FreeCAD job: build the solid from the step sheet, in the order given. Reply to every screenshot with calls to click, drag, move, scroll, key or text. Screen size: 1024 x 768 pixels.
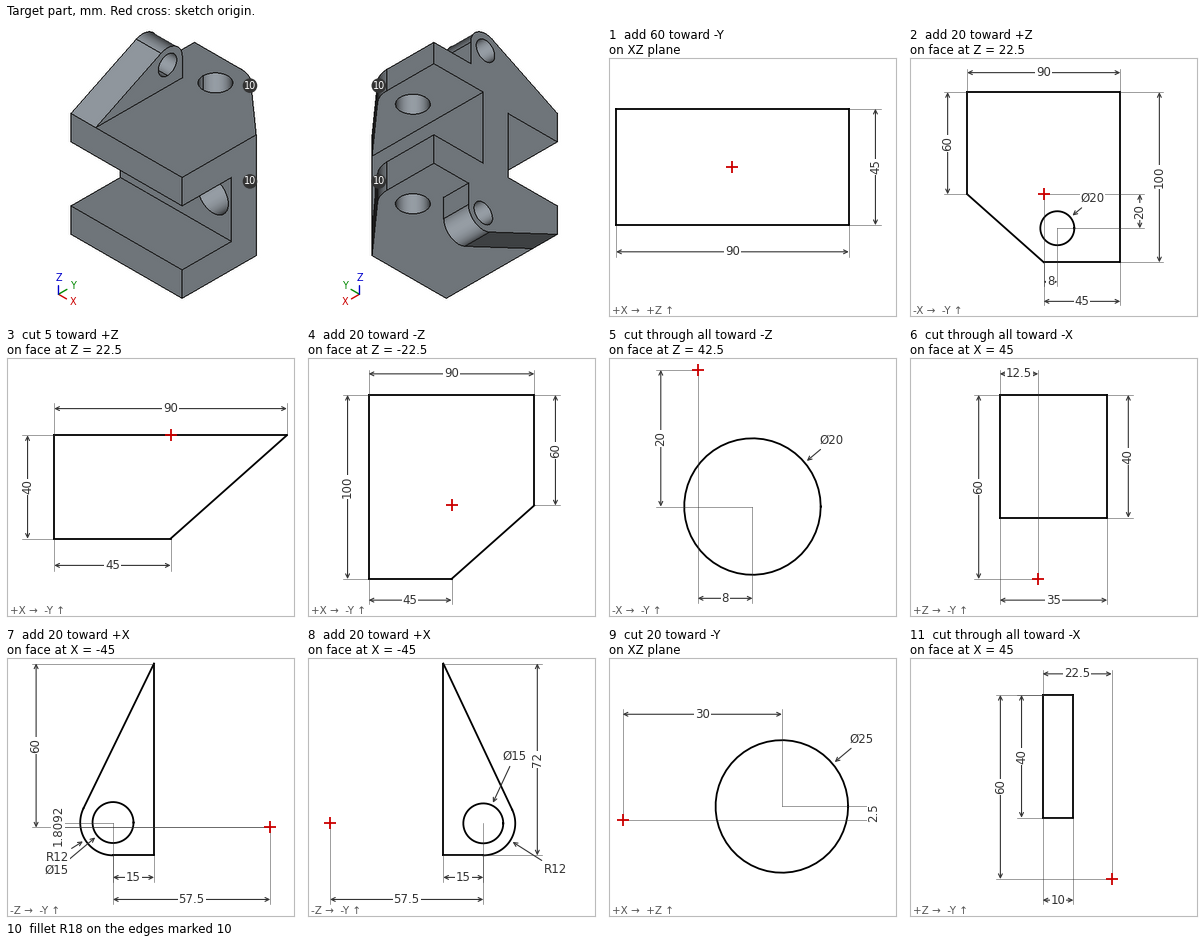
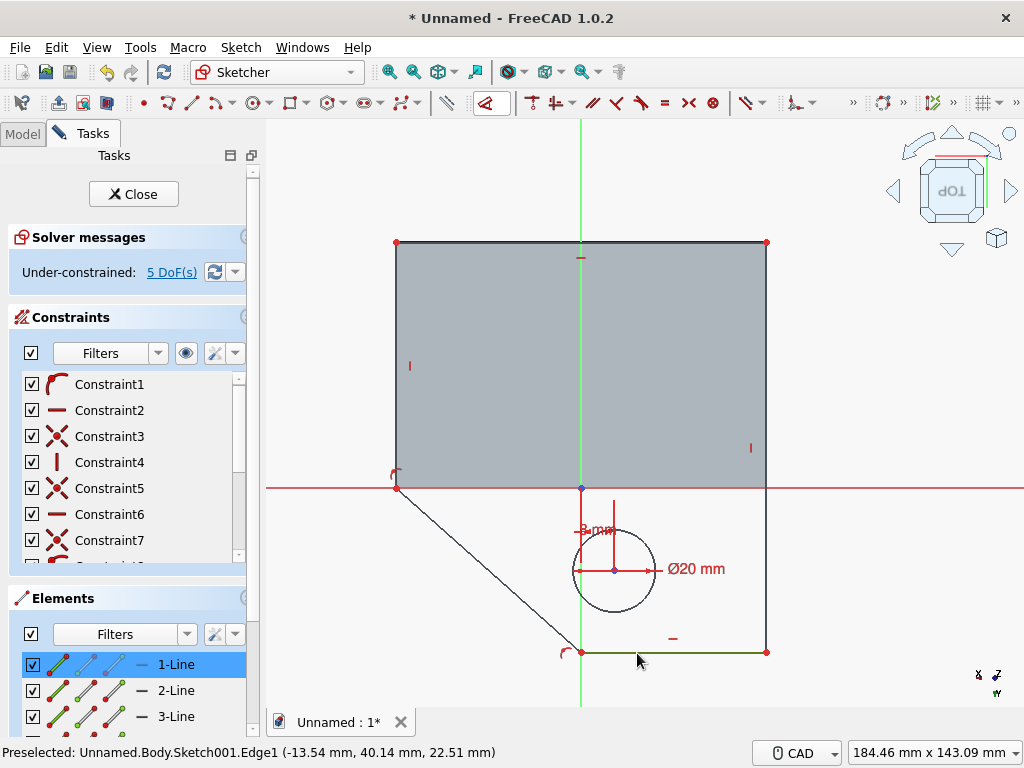
key(l)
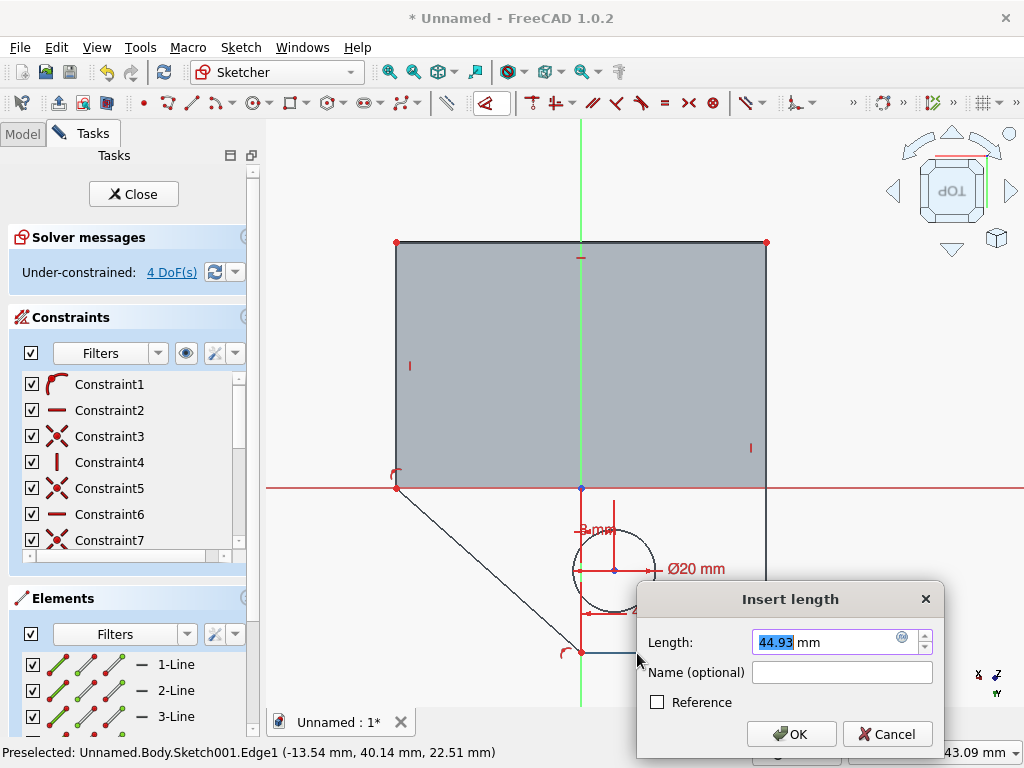
text(45)
key(Return)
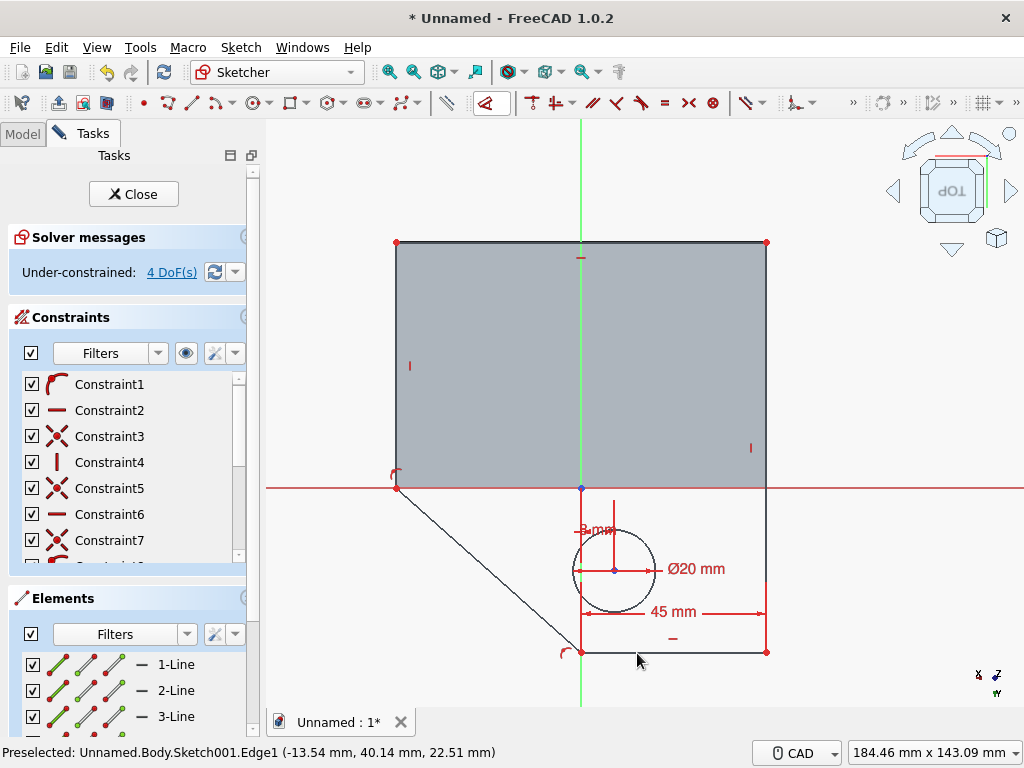
click(655, 243)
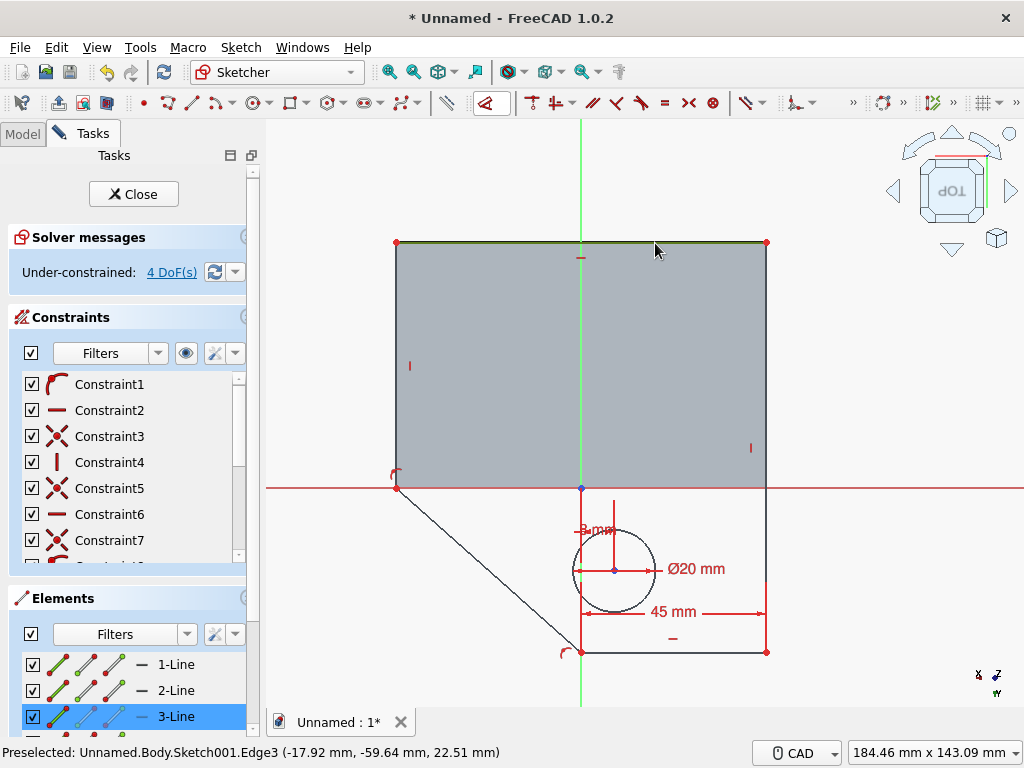
key(l)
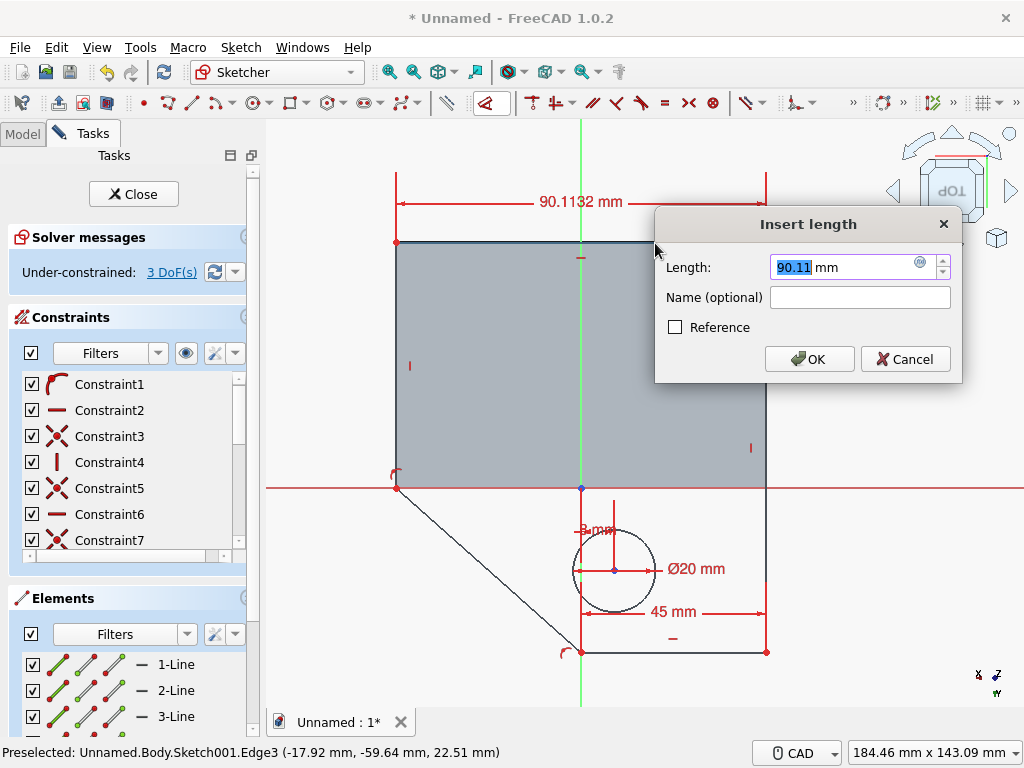
text(90)
key(Return)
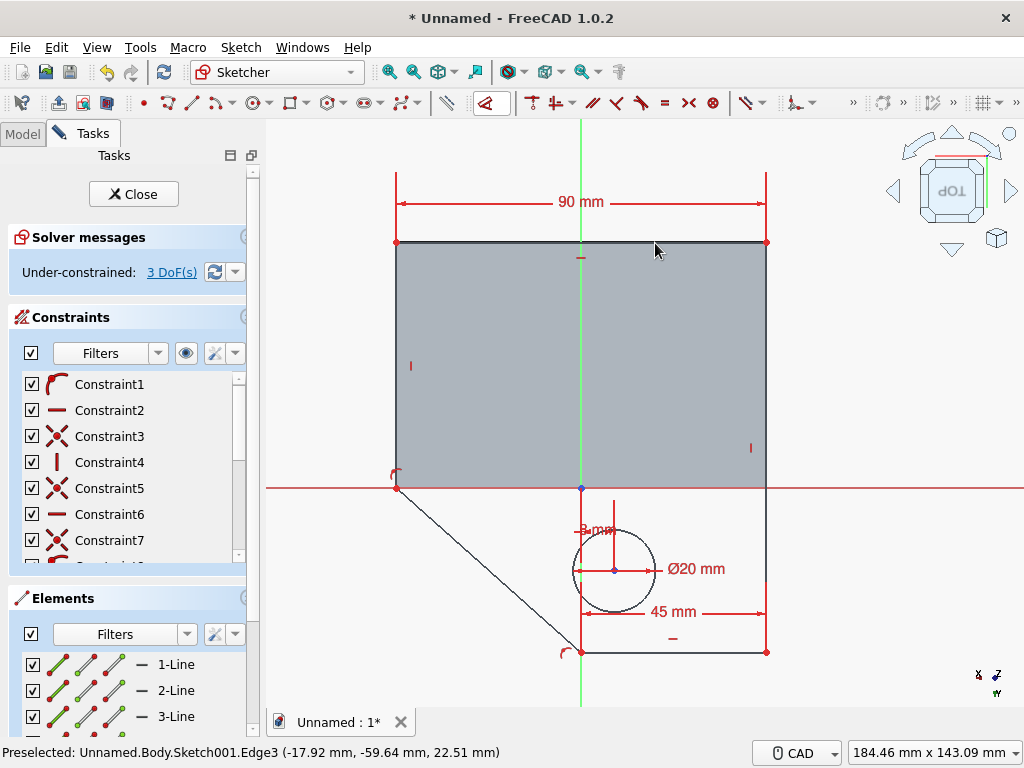
click(396, 317)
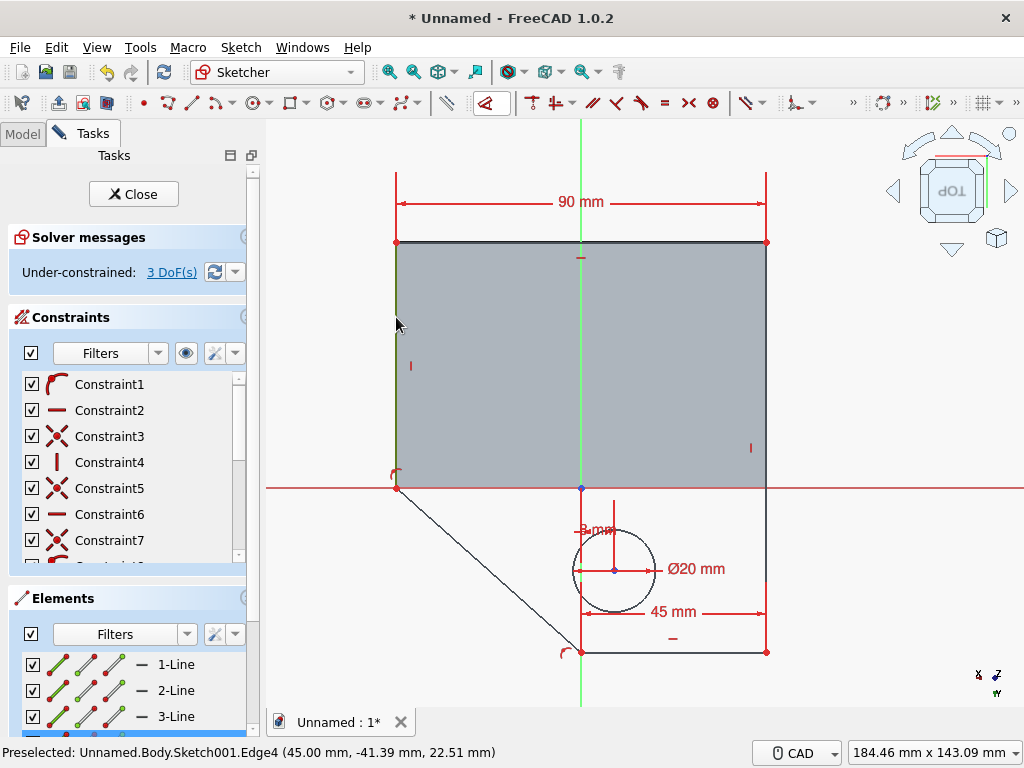
key(i)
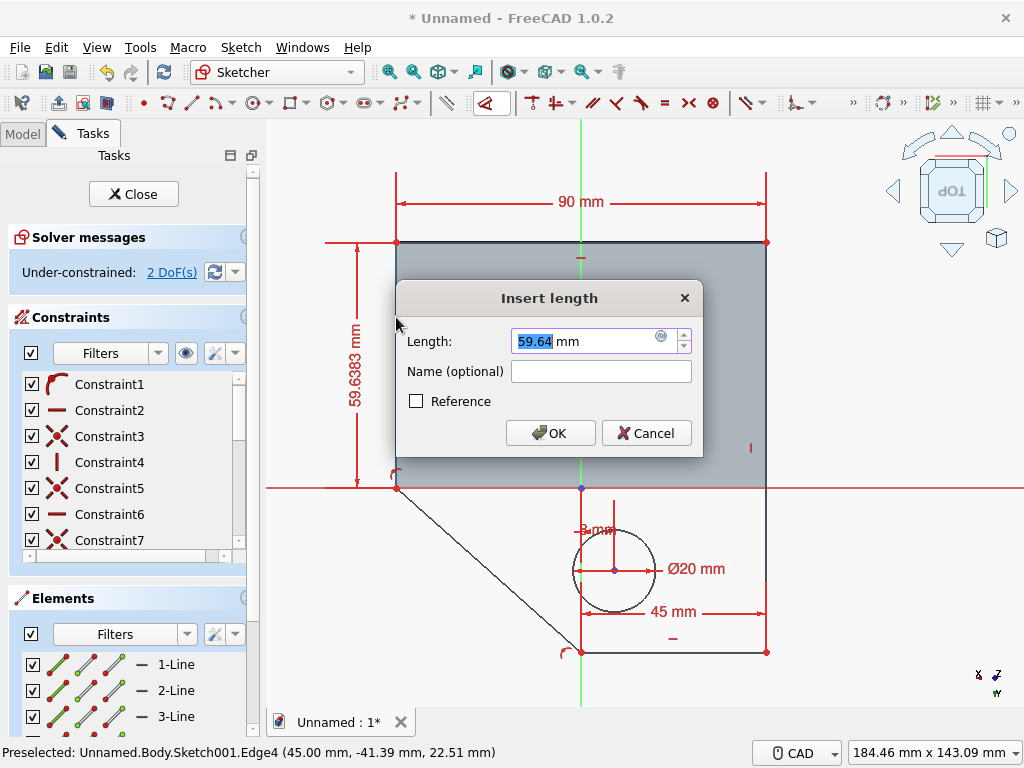
text(60)
key(Return)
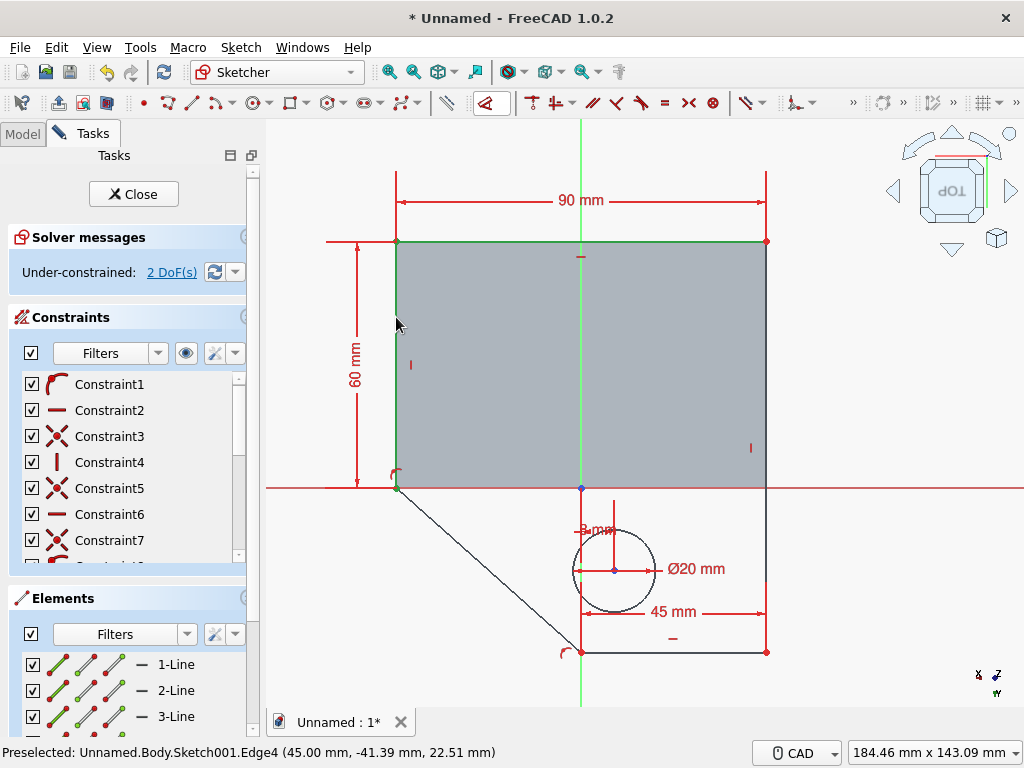
click(614, 571)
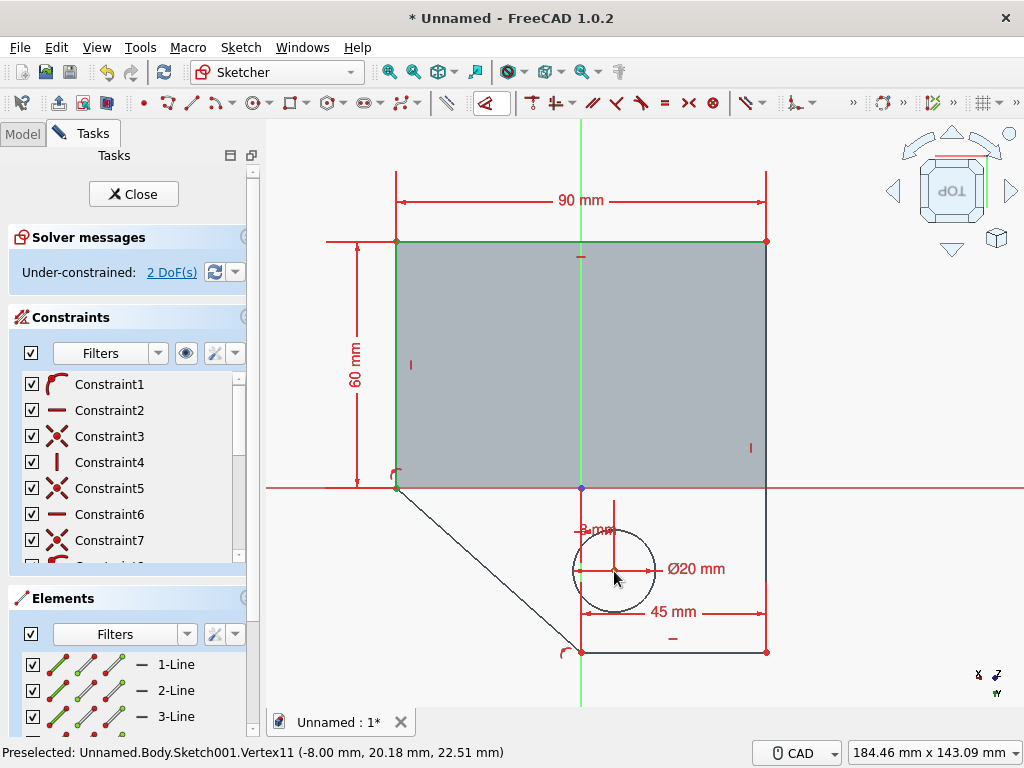
key(i)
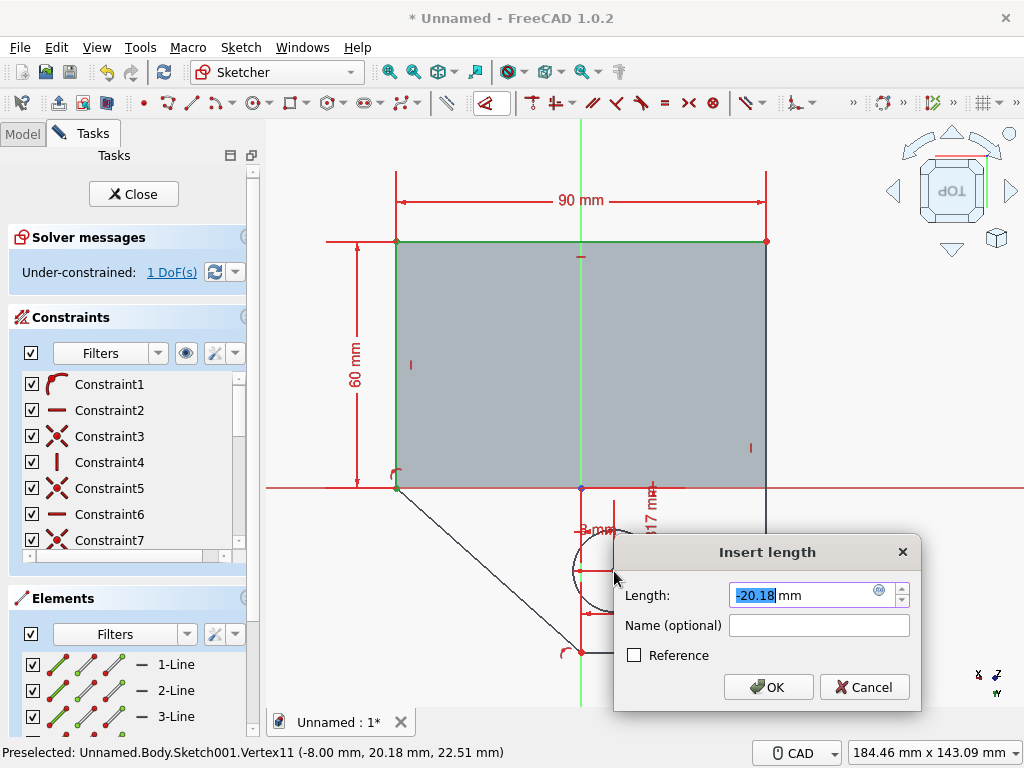
text(-20)
key(Return)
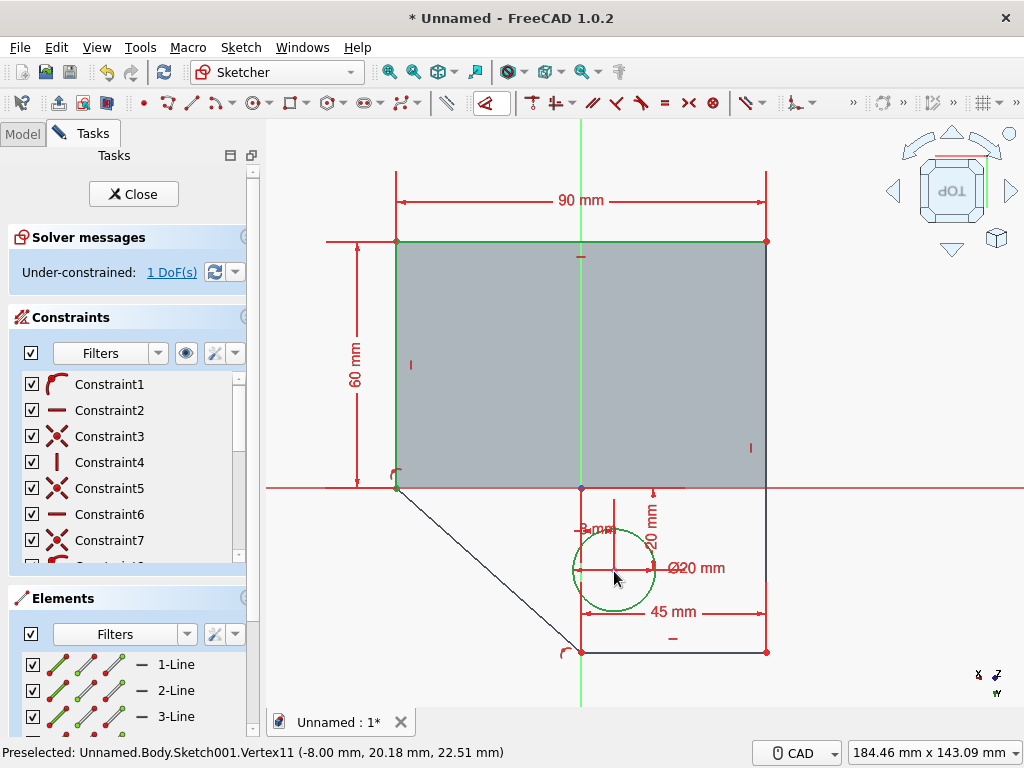
click(766, 530)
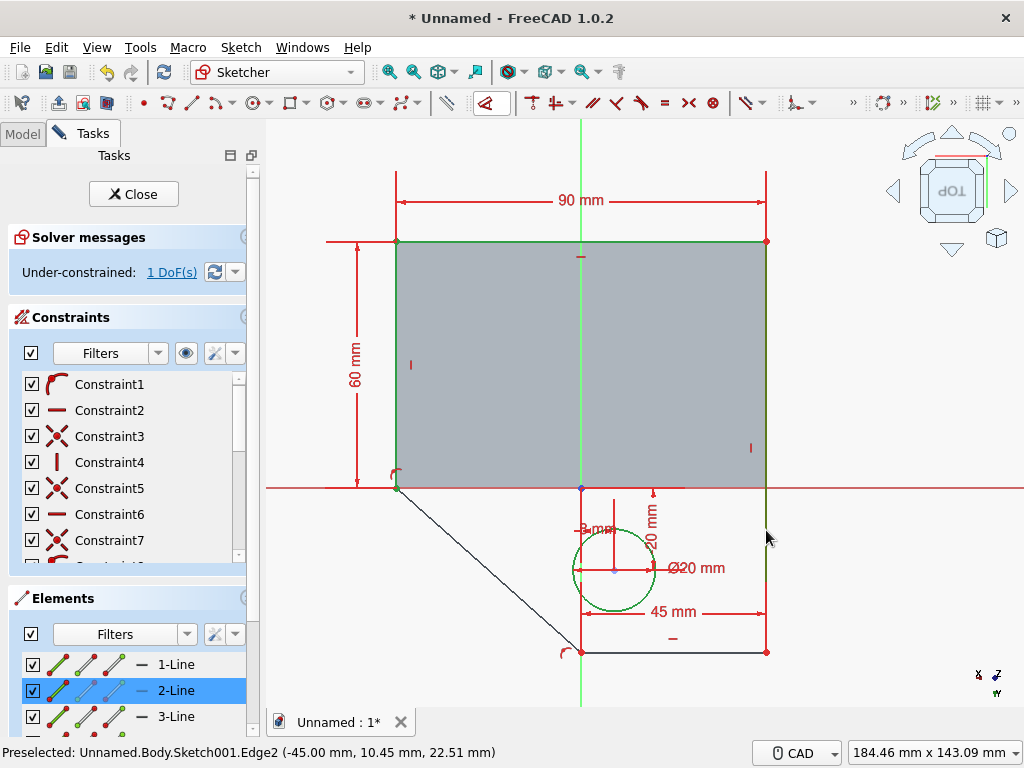
click(504, 104)